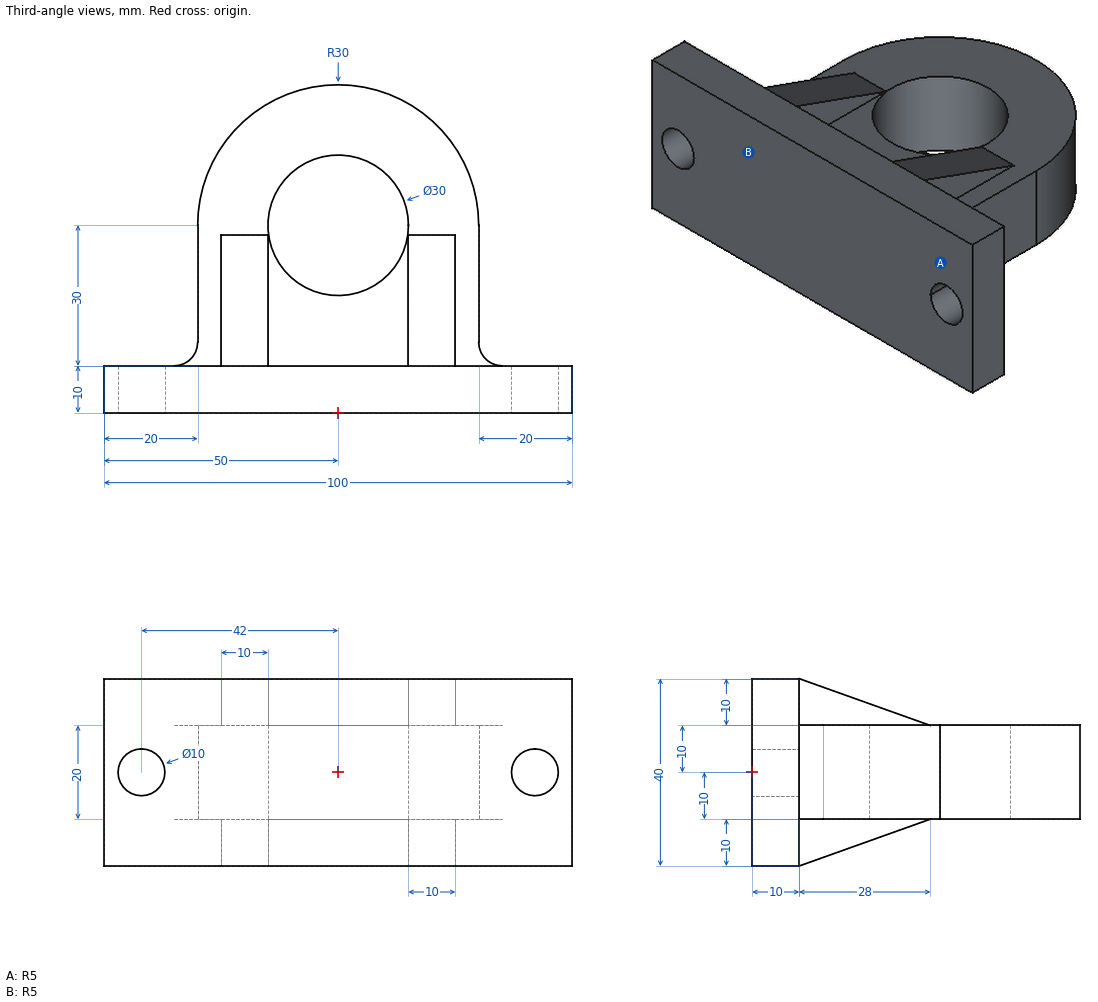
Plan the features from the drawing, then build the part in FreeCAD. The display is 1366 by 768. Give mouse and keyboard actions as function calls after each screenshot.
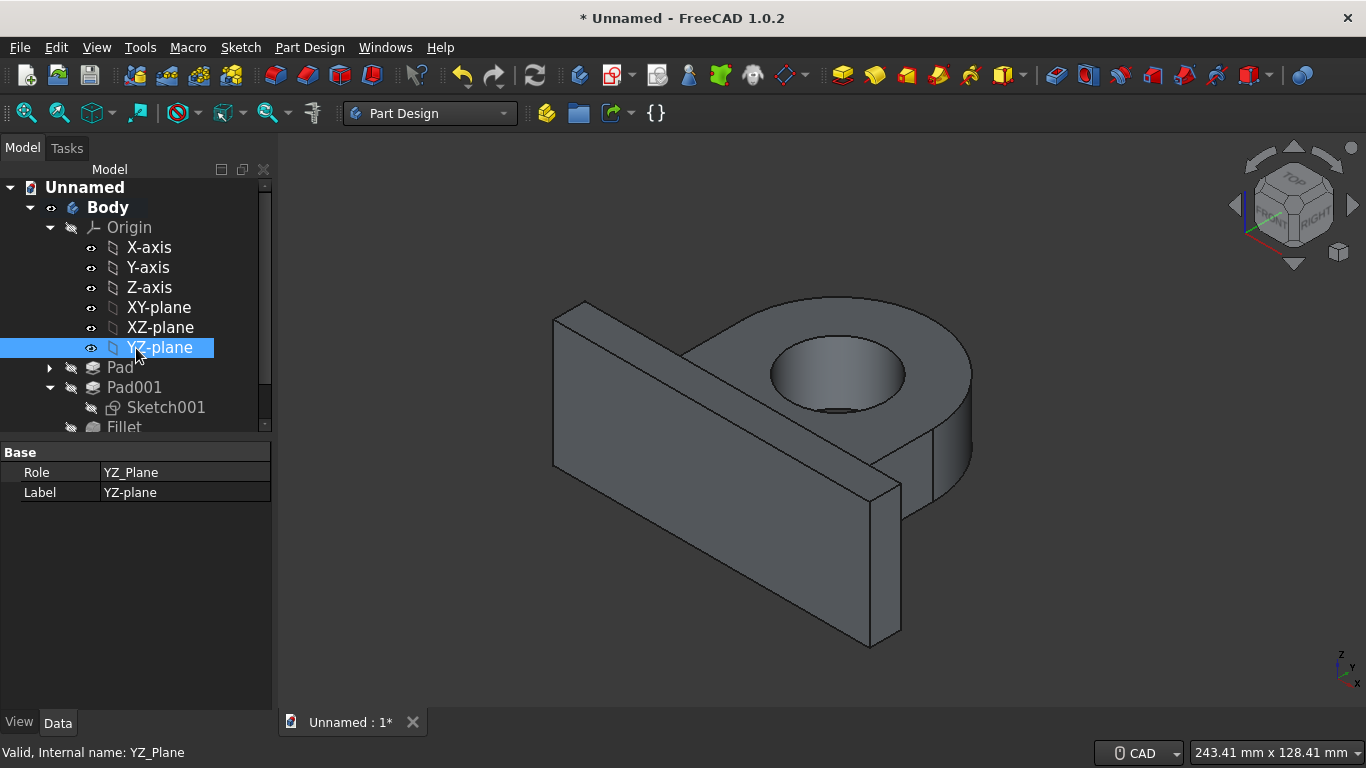
click(786, 76)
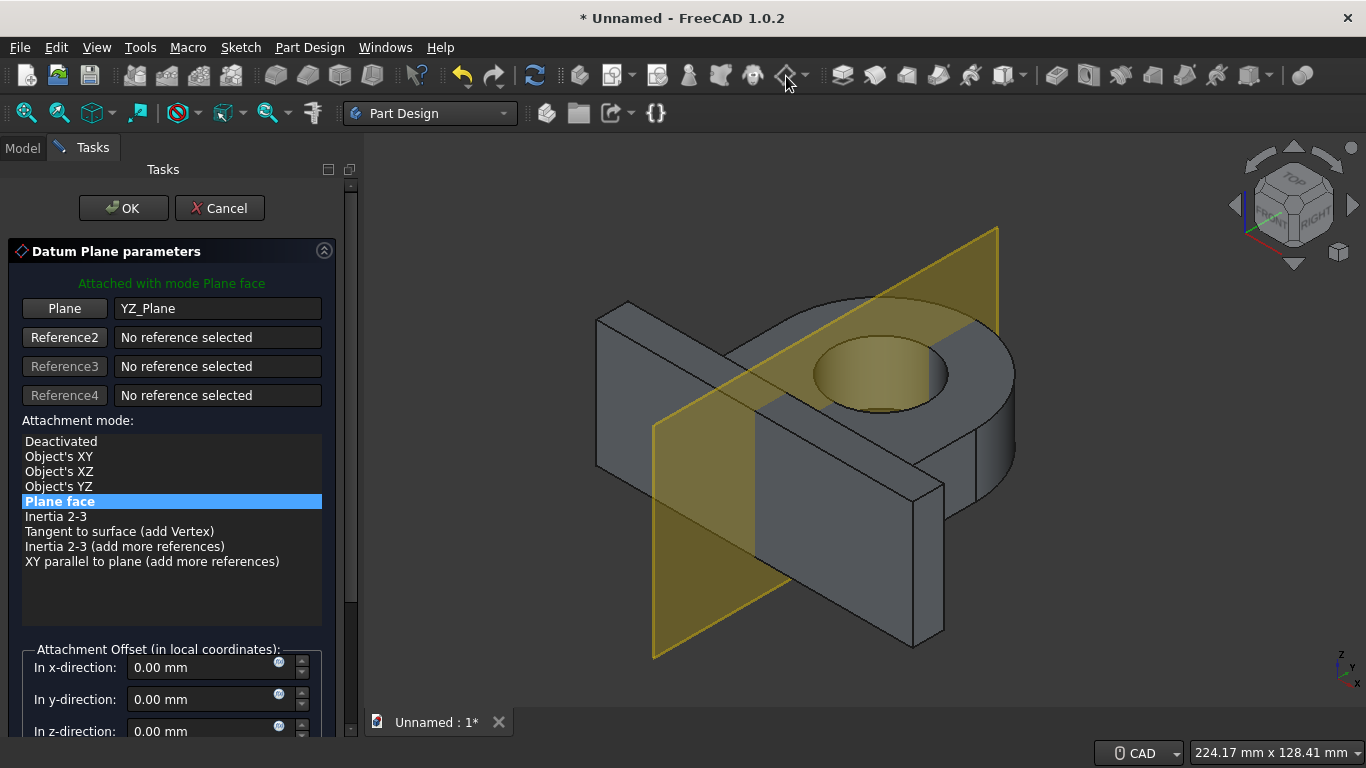
scroll(351, 458, down, 2)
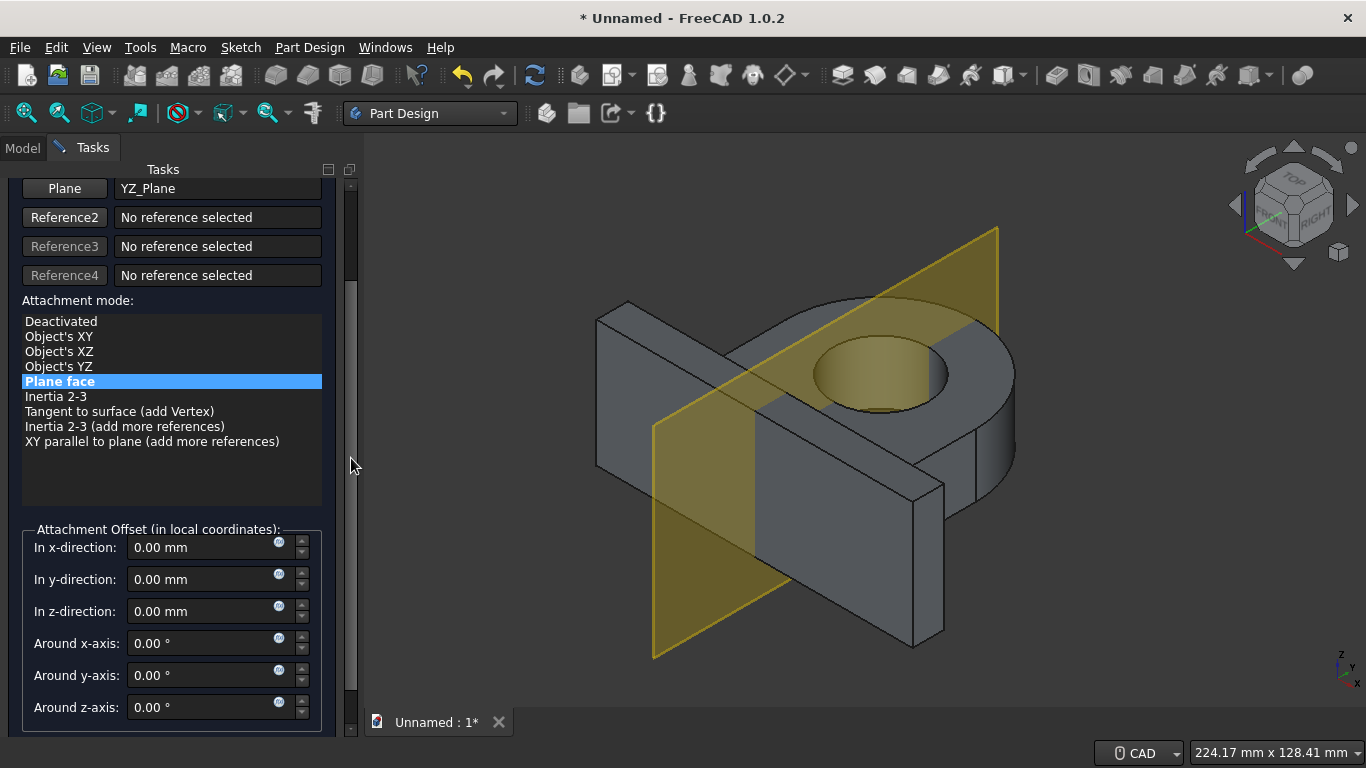
triple_click(210, 611)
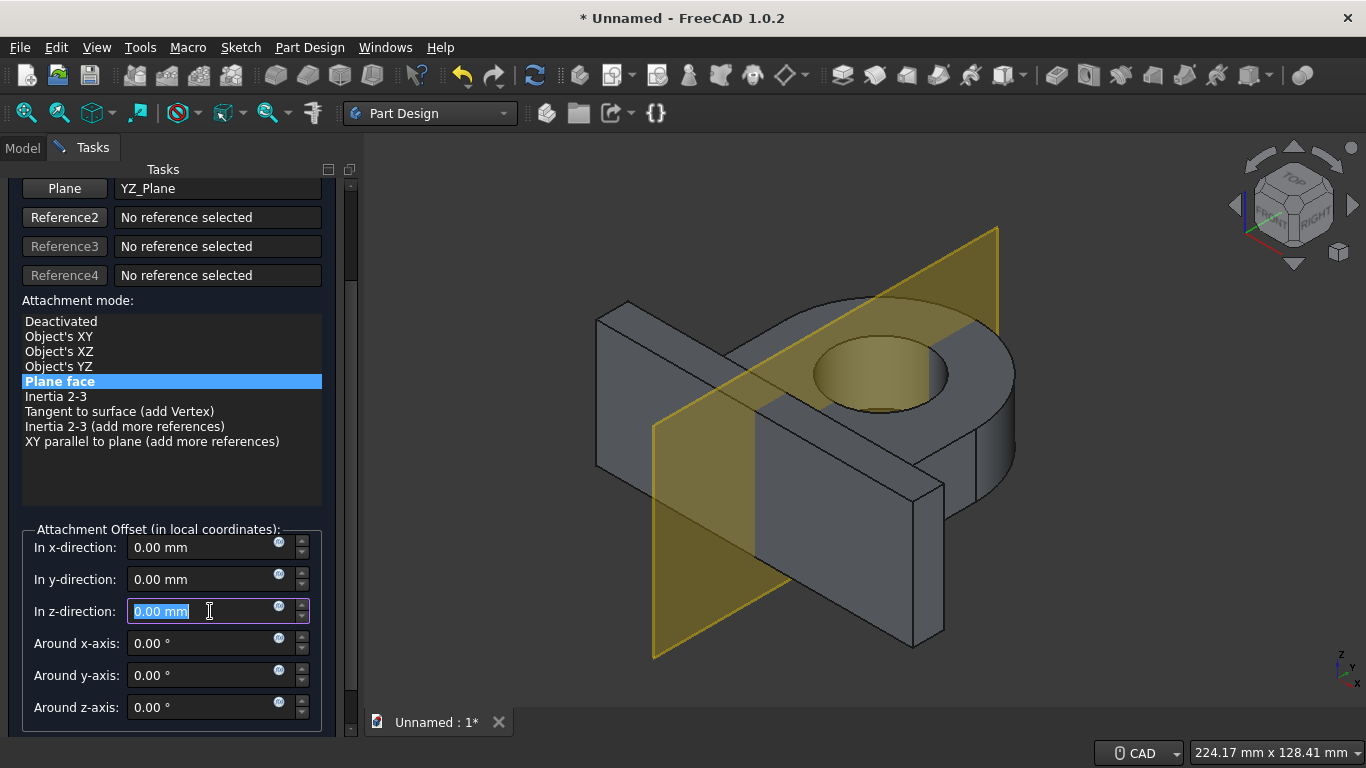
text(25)
key(Tab)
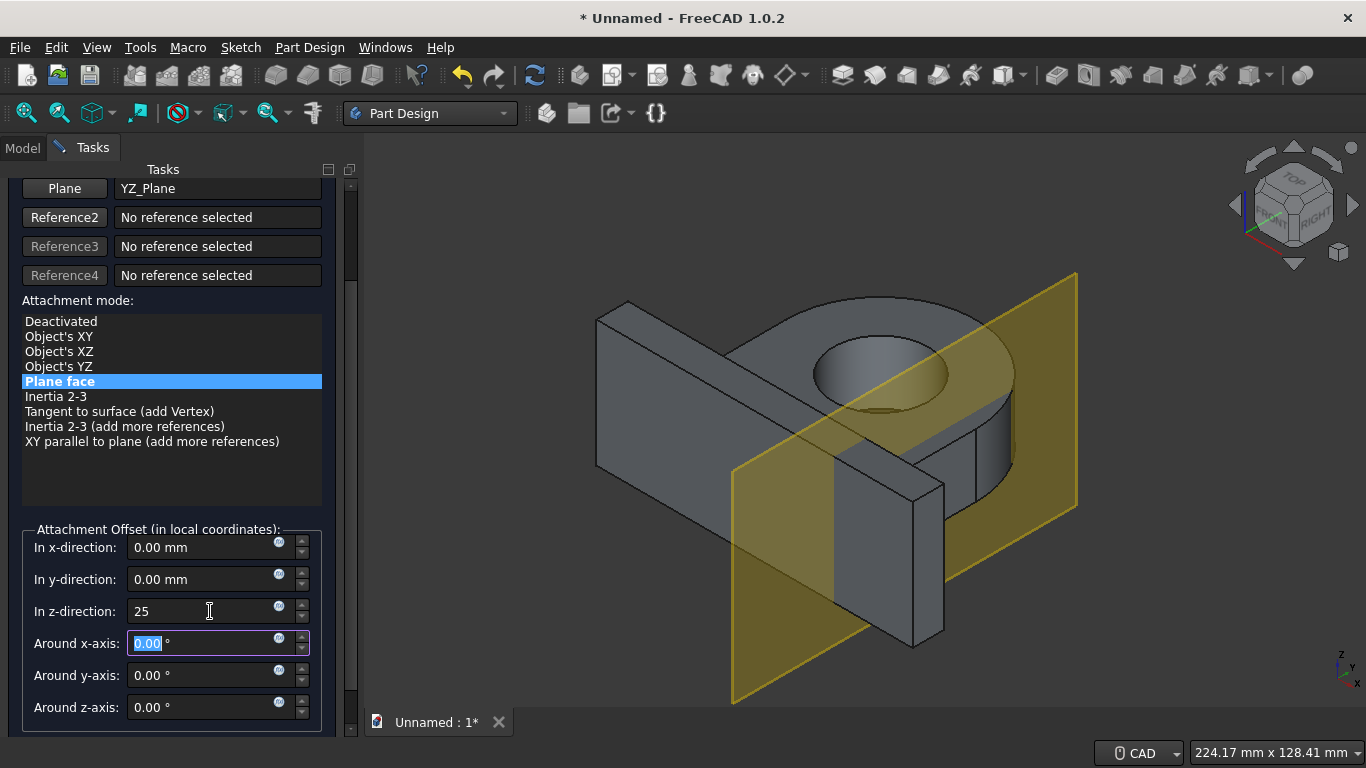
scroll(351, 458, up, 3)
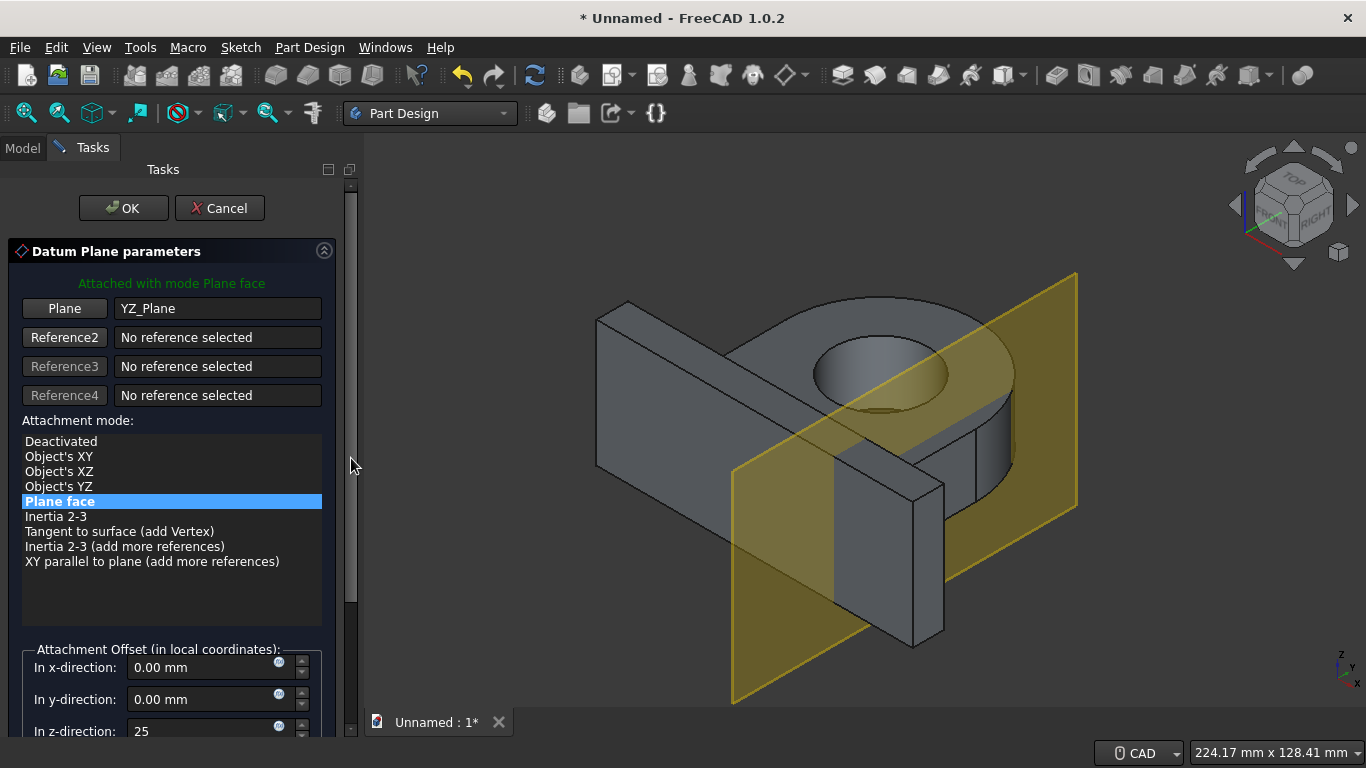
click(124, 208)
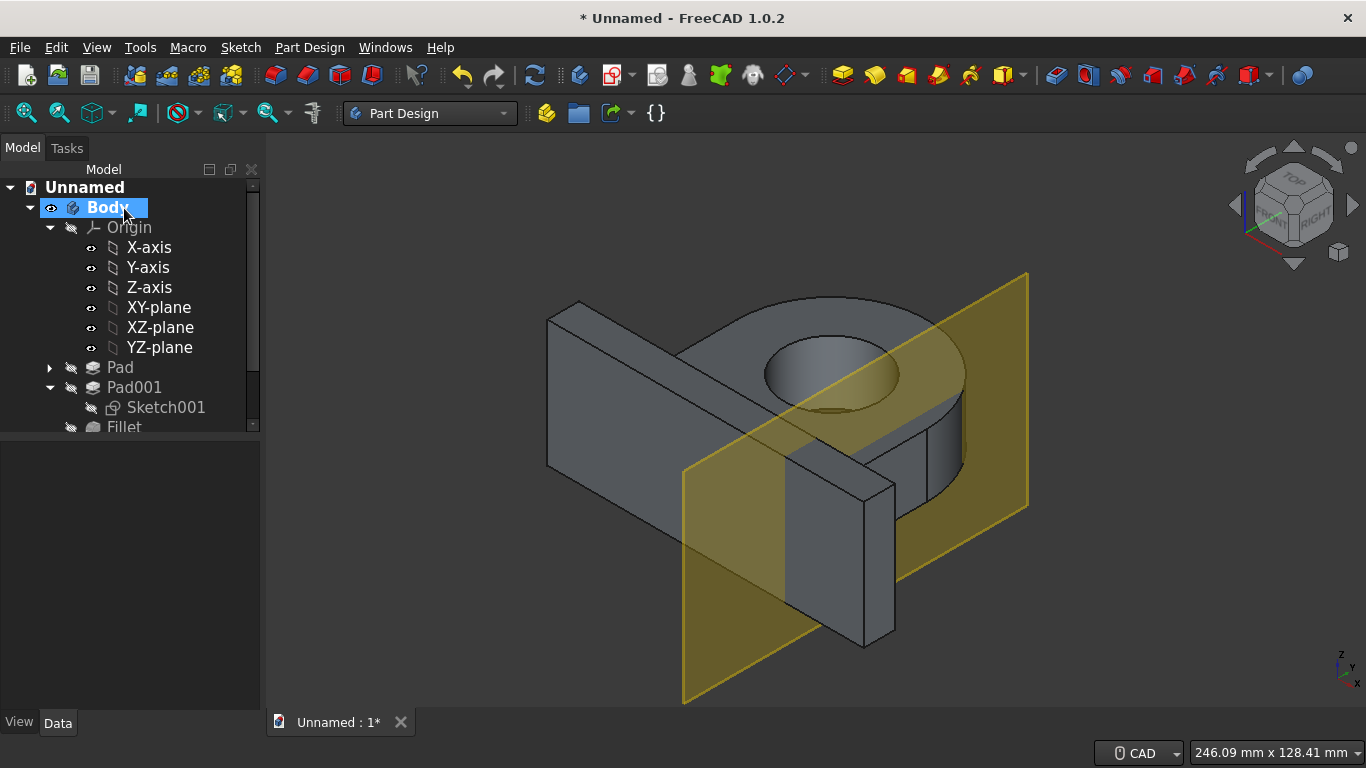
scroll(100, 303, down, 3)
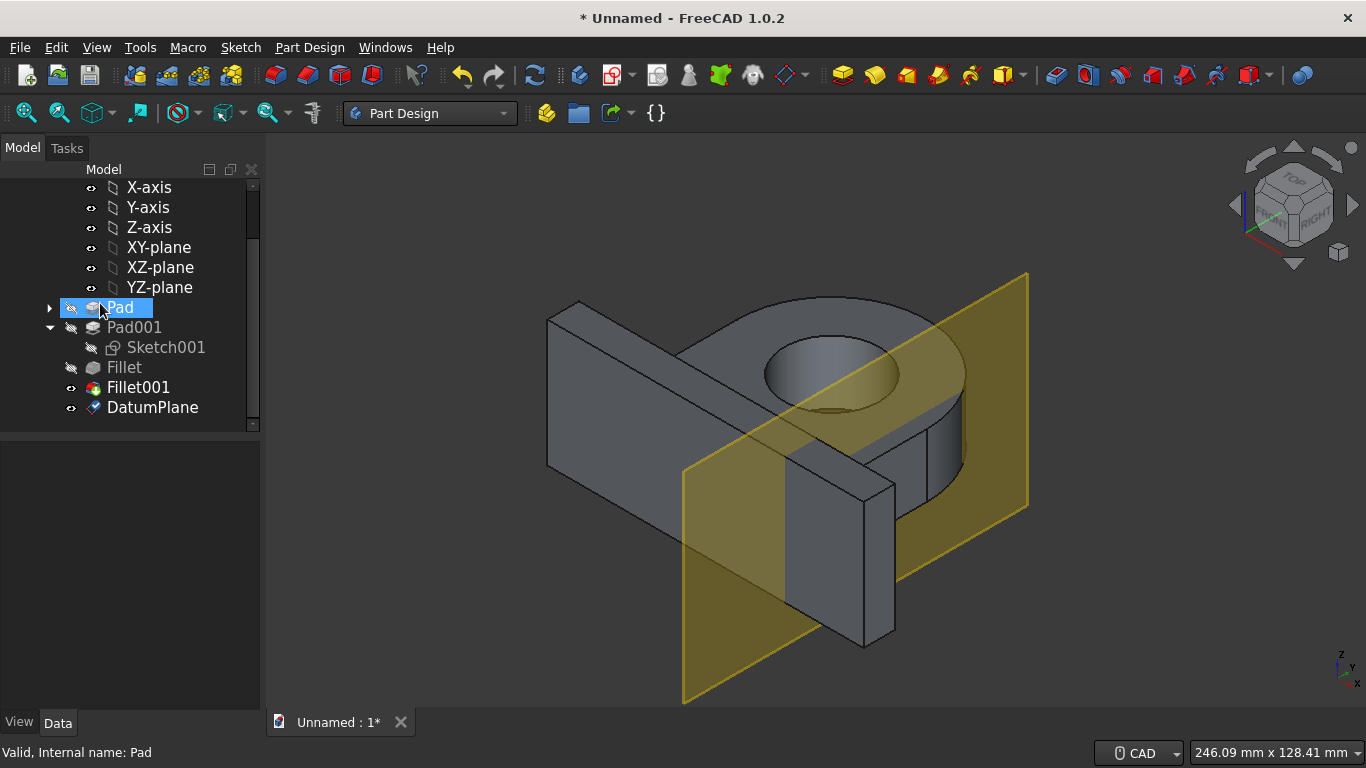
click(116, 408)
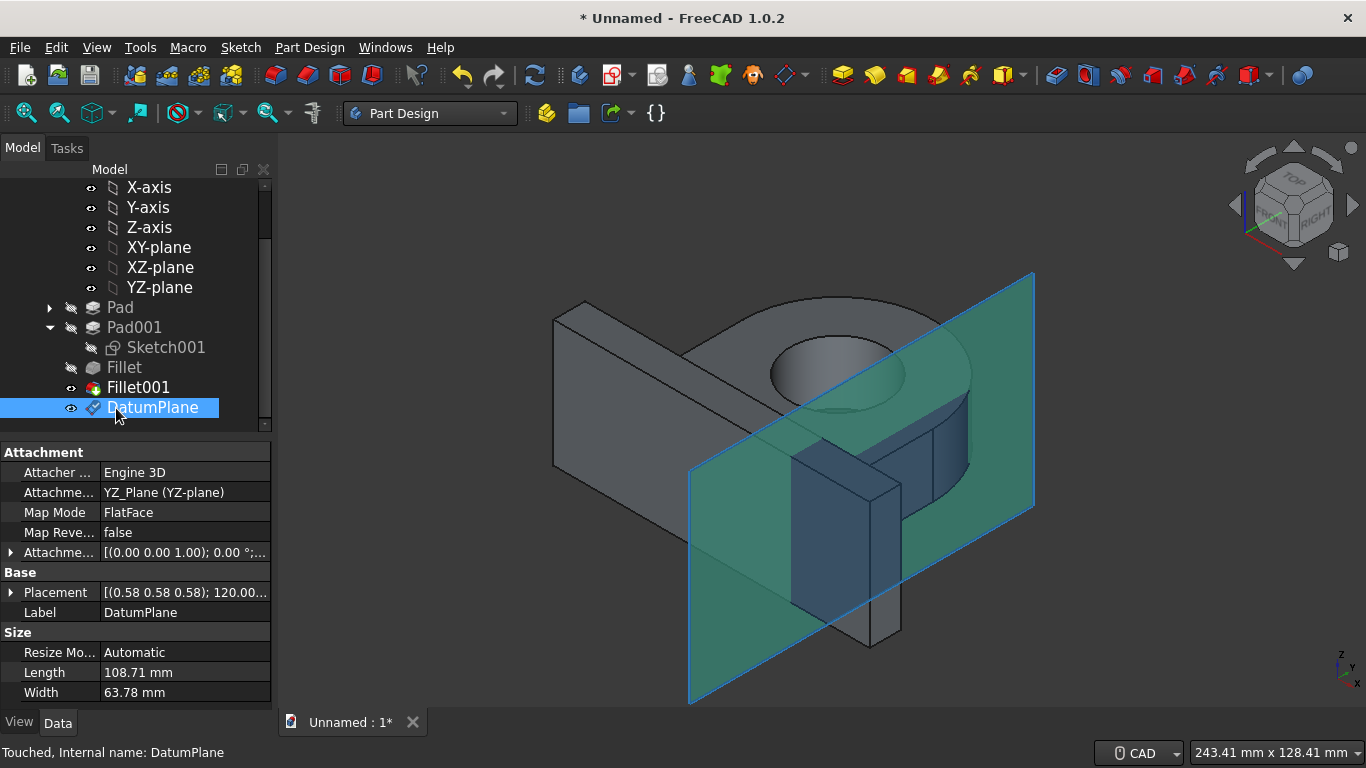
click(612, 76)